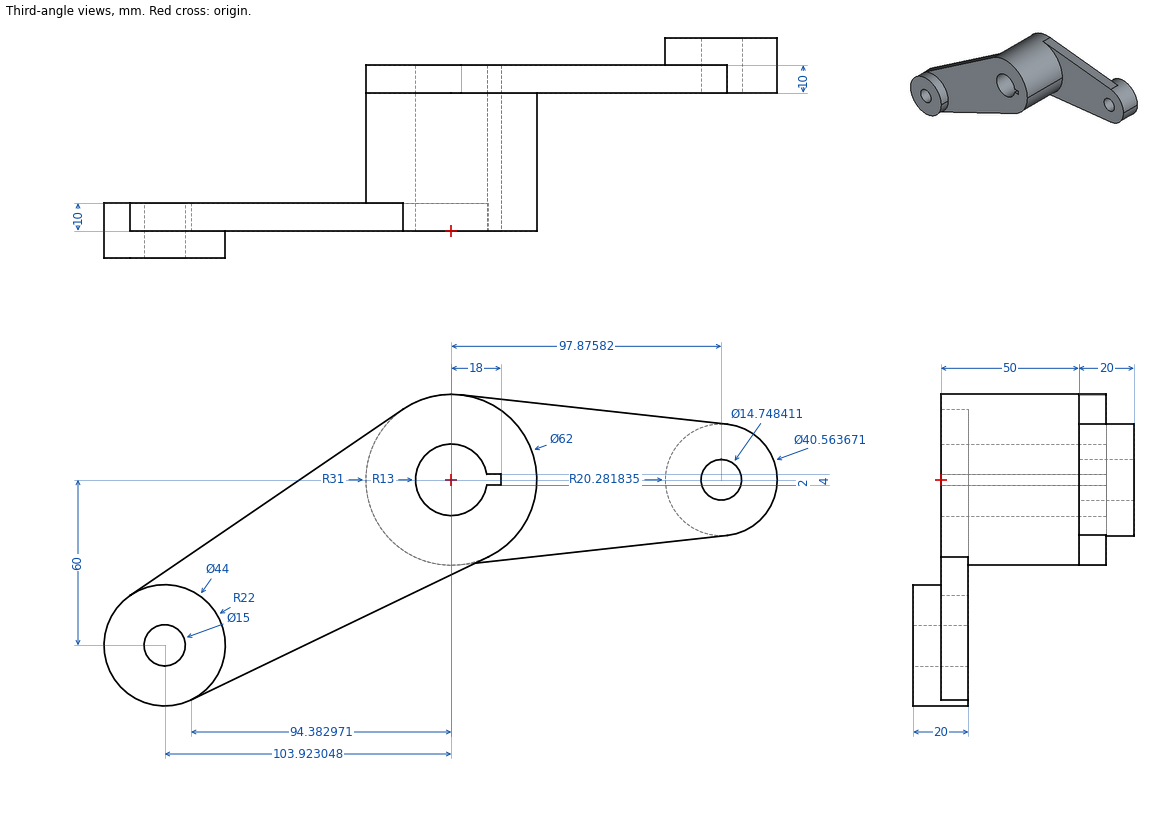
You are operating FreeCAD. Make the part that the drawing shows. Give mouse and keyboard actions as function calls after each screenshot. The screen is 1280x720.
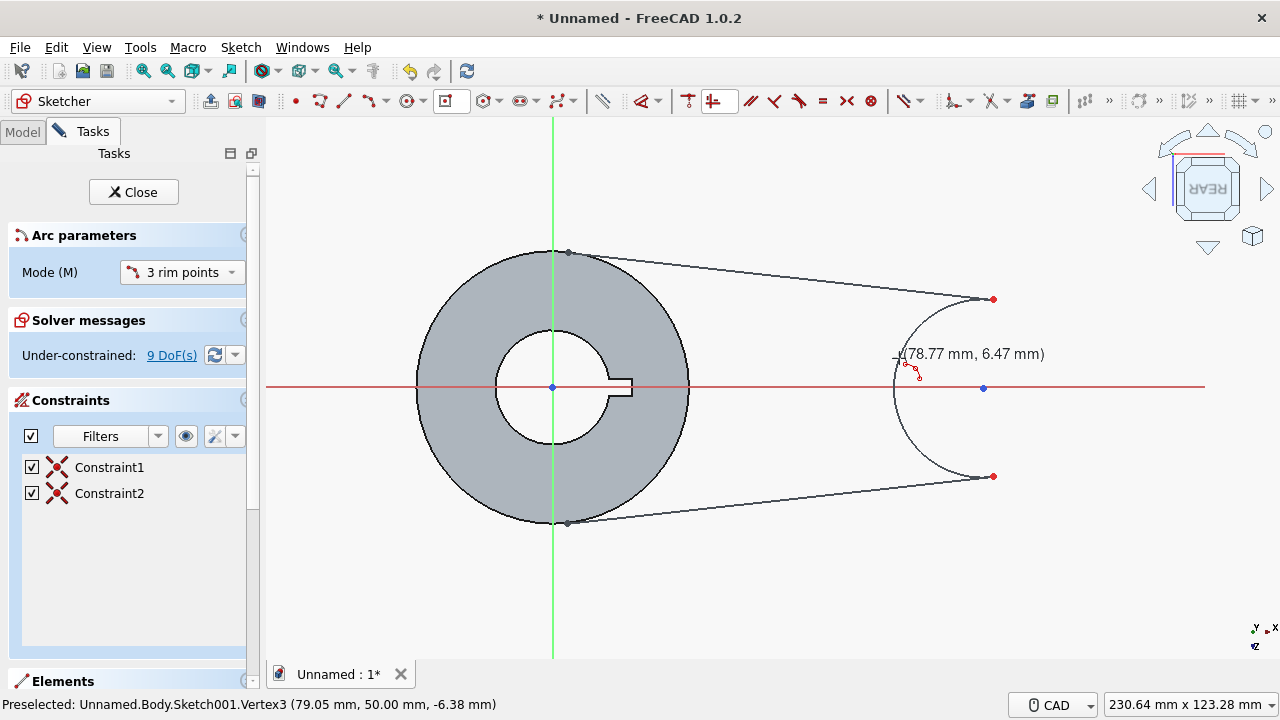
click(568, 253)
click(567, 524)
click(424, 342)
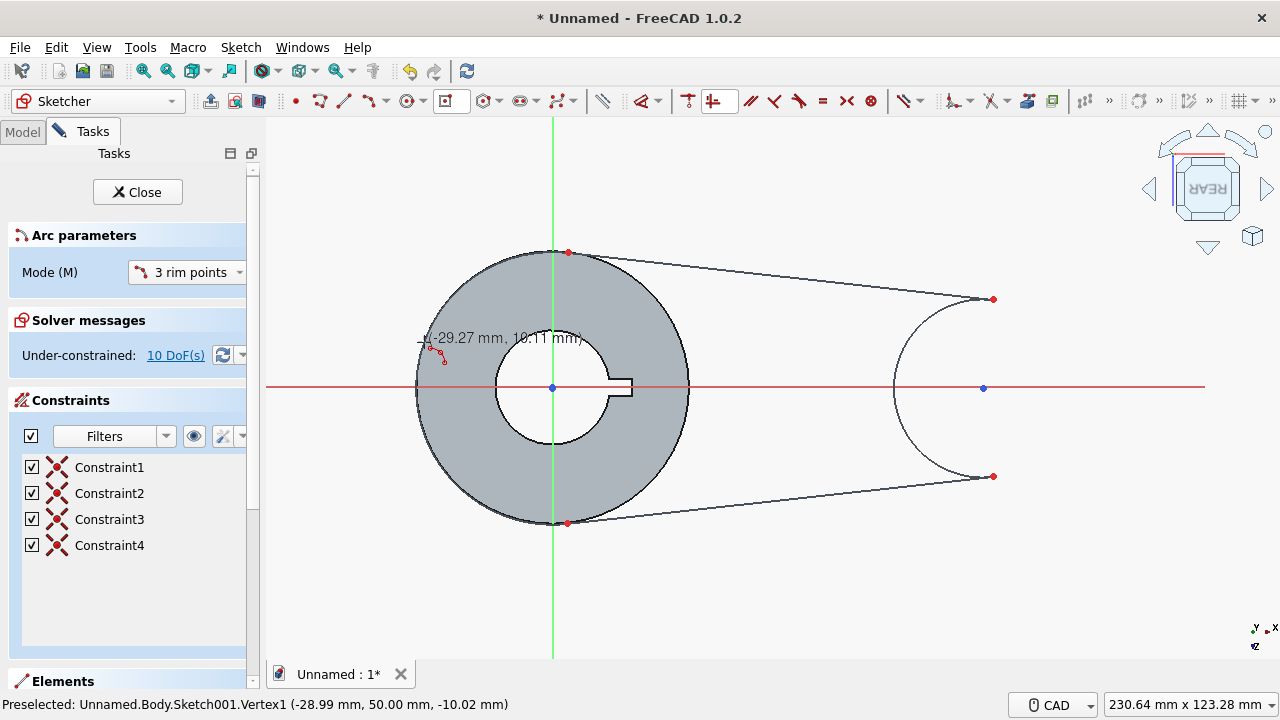
click(320, 102)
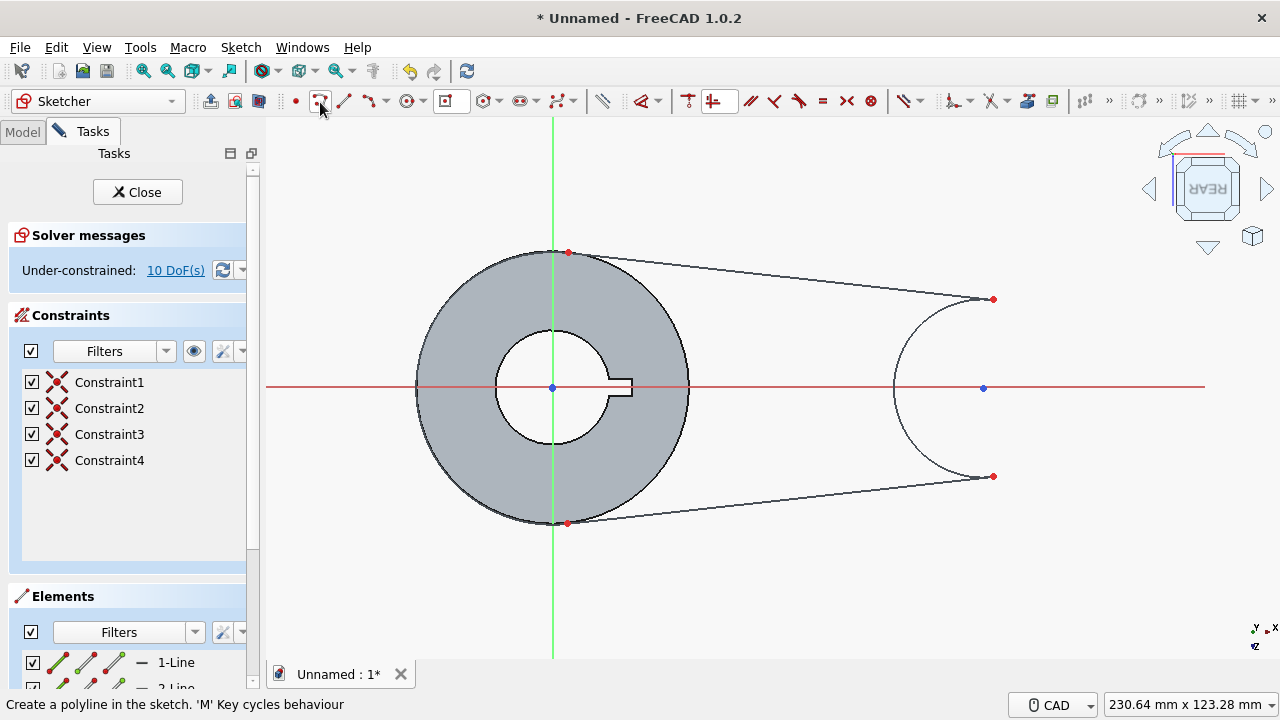
scroll(609, 379, up, 3)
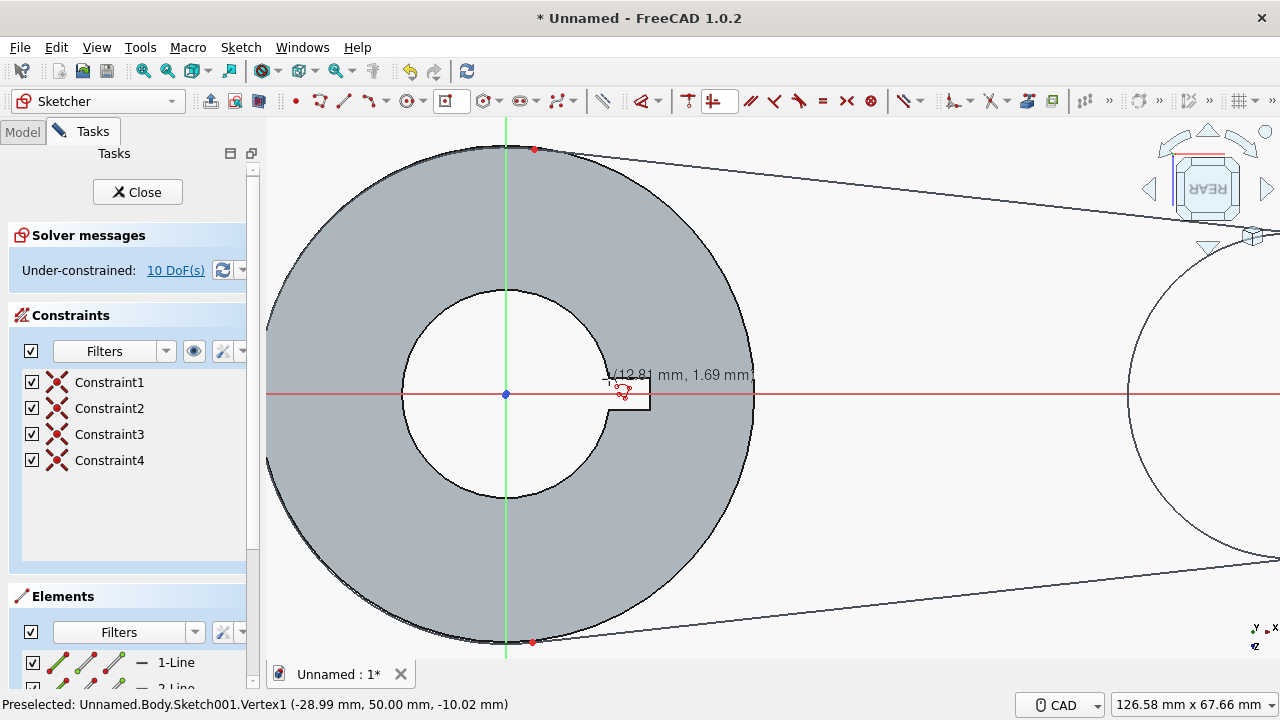
click(609, 378)
click(650, 378)
click(650, 410)
click(609, 410)
right_click(609, 410)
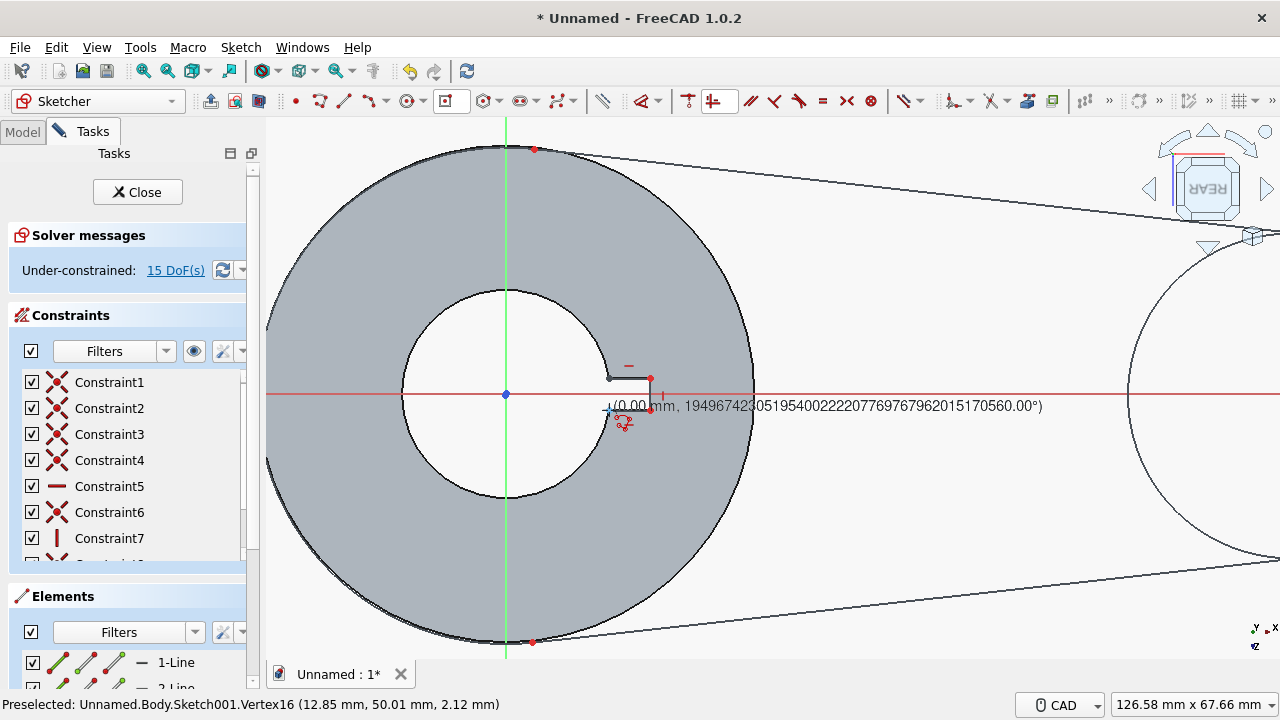
click(370, 102)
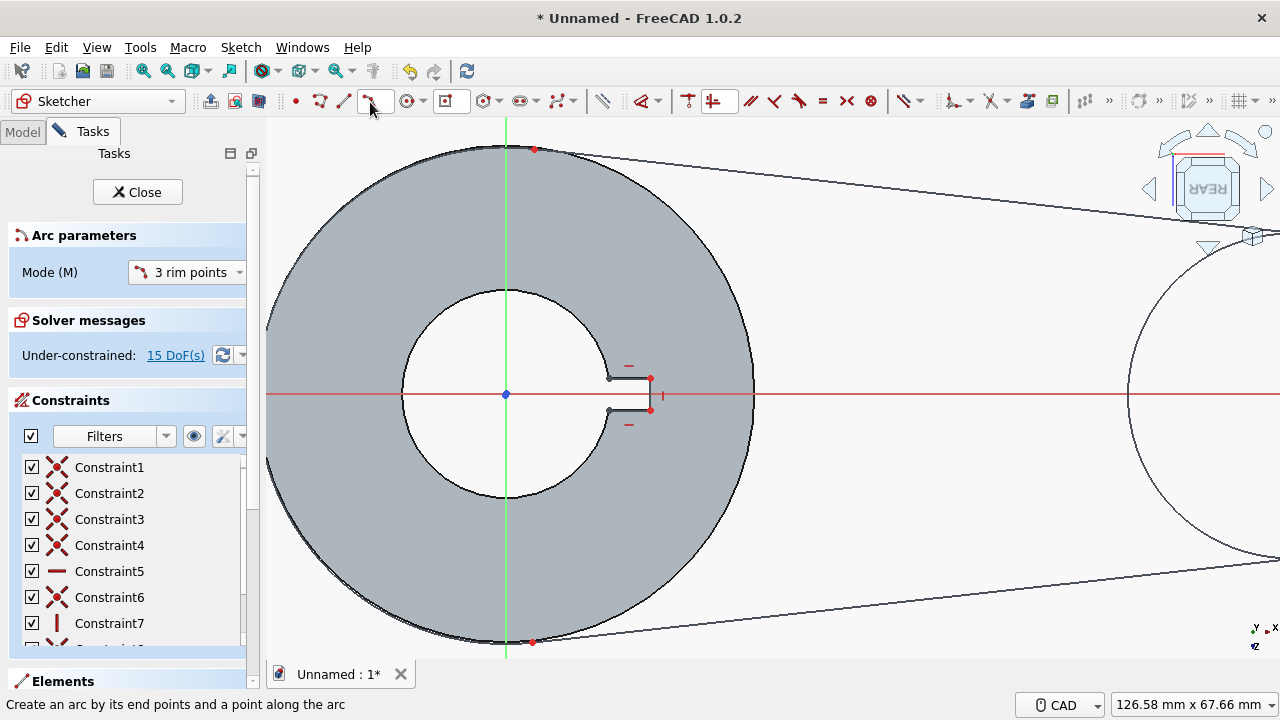
click(609, 411)
click(609, 379)
click(420, 335)
key(Escape)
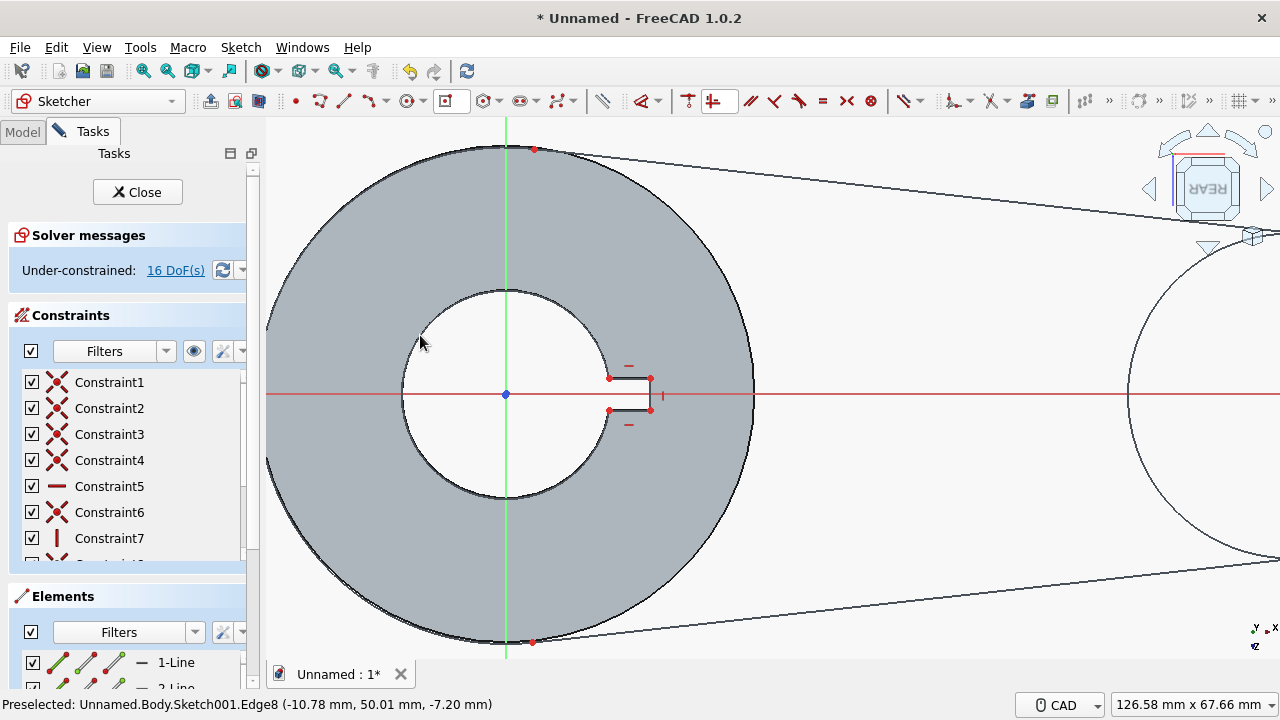
click(766, 617)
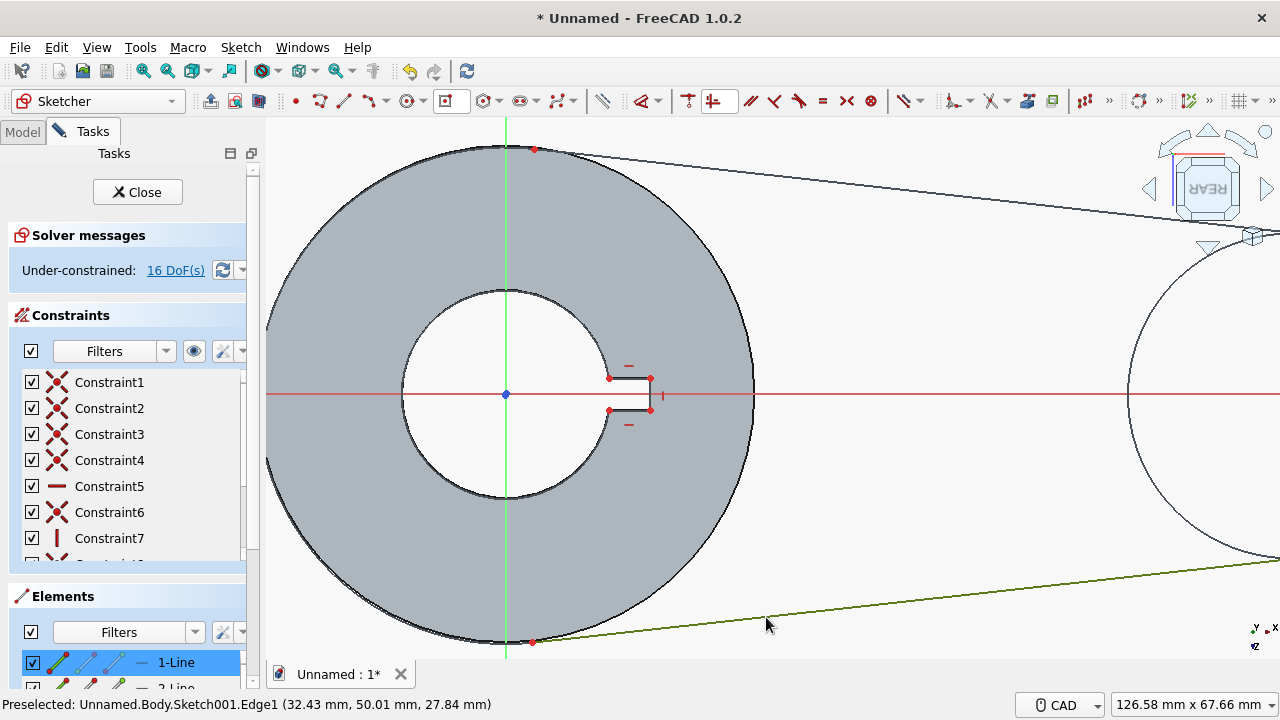
scroll(609, 381, down, 3)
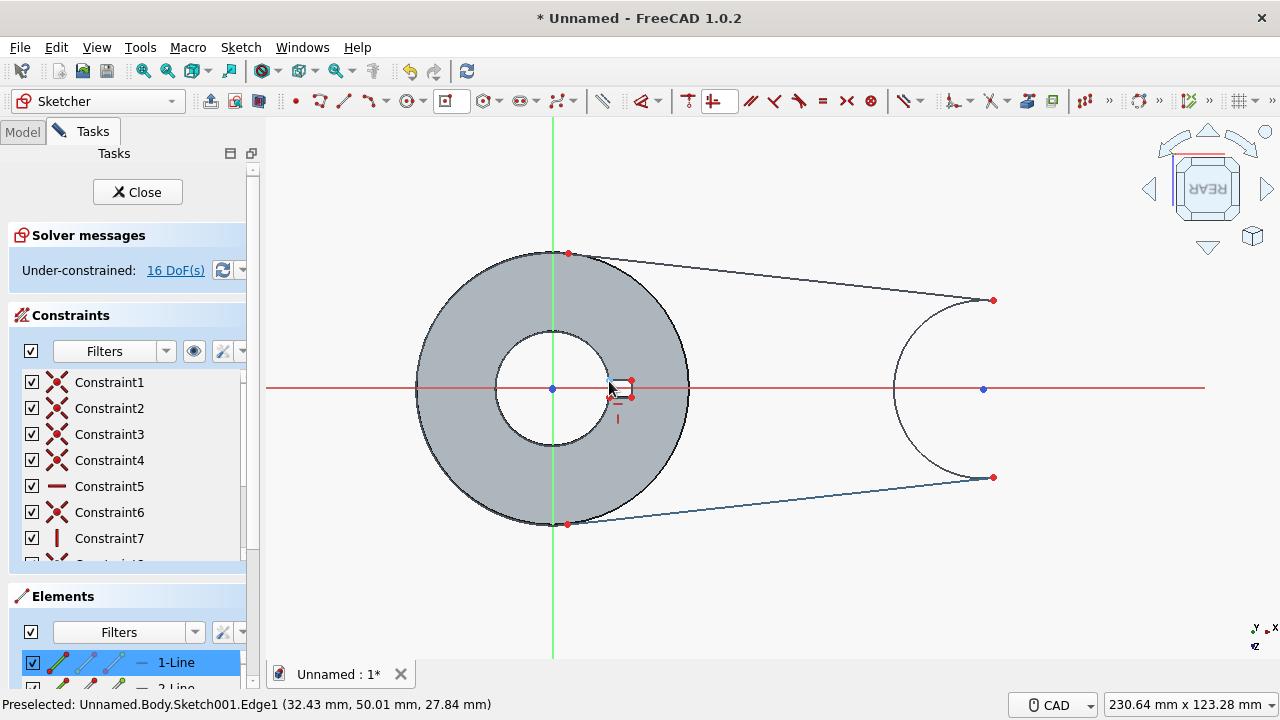
click(913, 334)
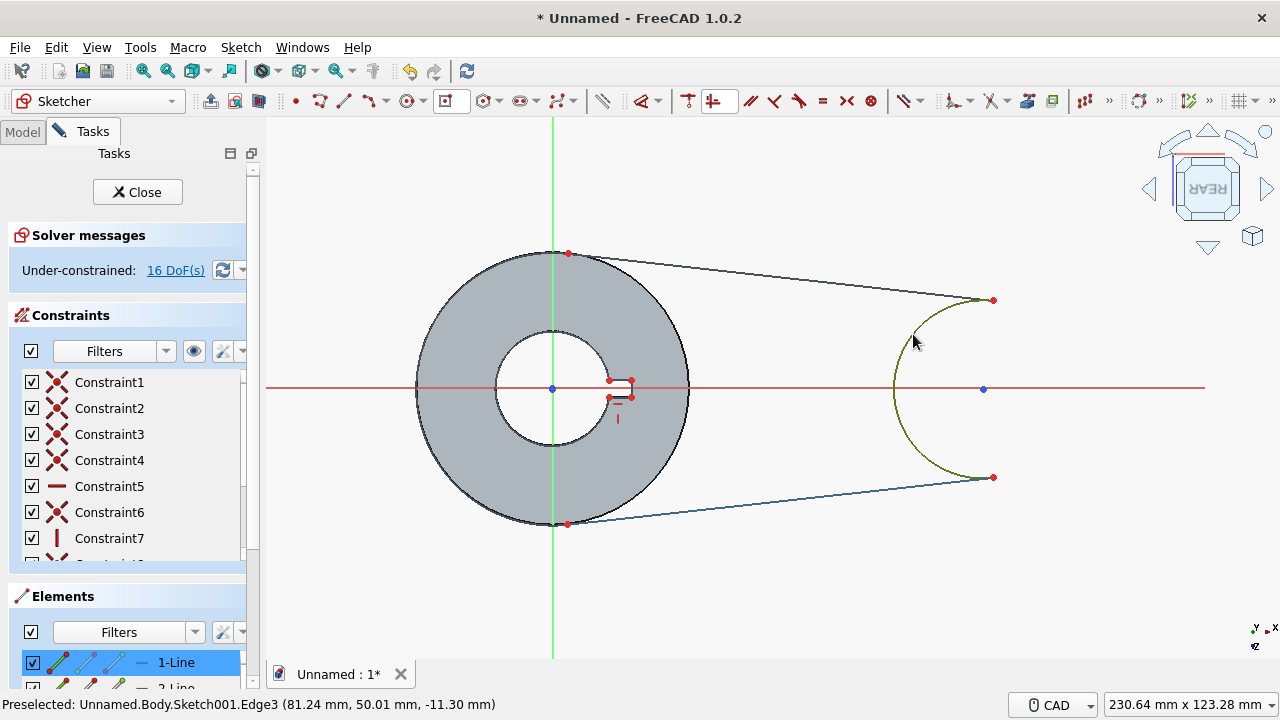
key(t)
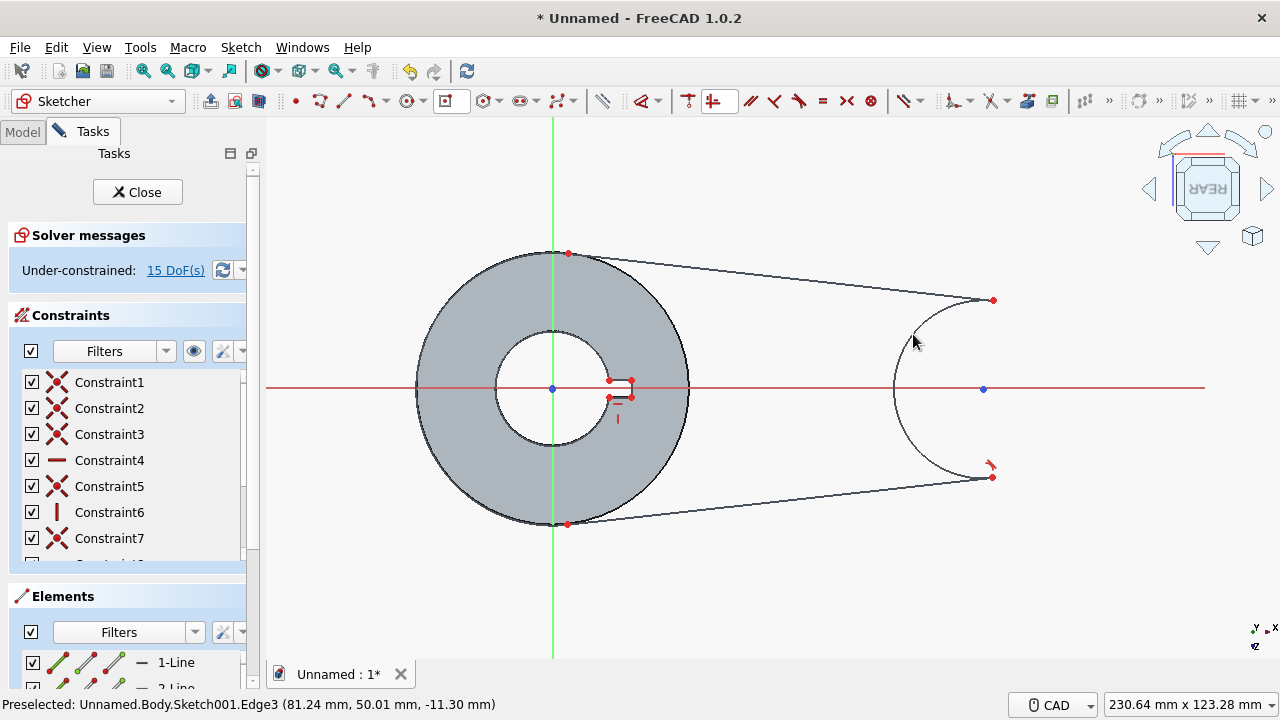
click(695, 511)